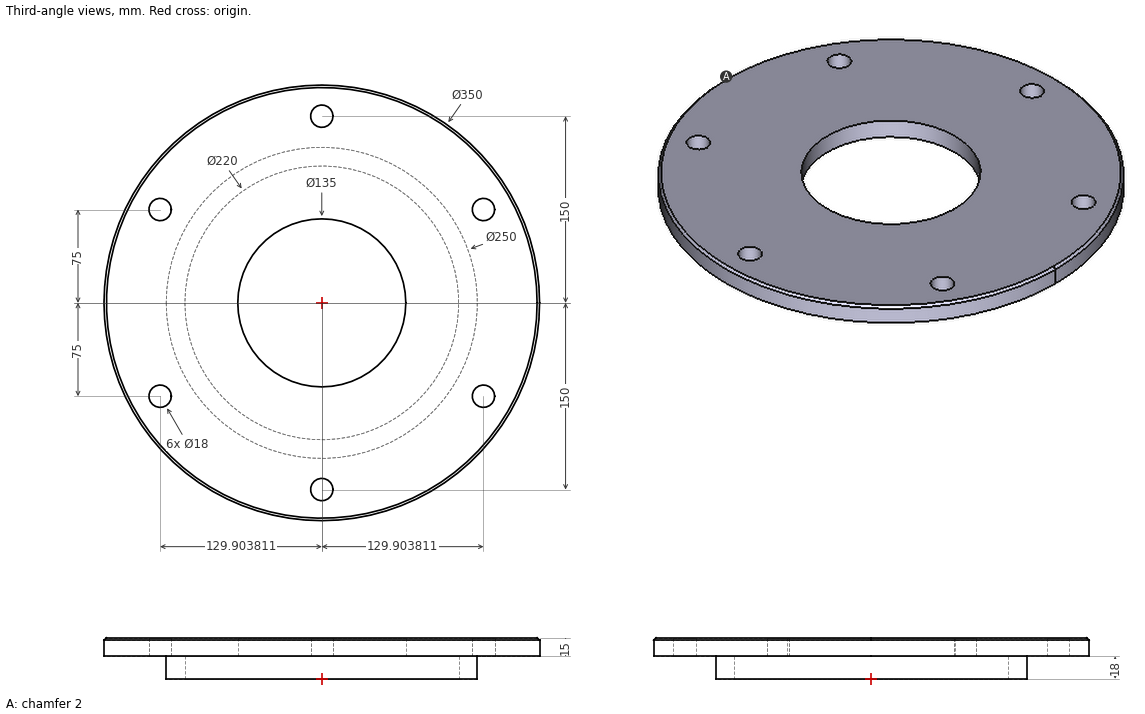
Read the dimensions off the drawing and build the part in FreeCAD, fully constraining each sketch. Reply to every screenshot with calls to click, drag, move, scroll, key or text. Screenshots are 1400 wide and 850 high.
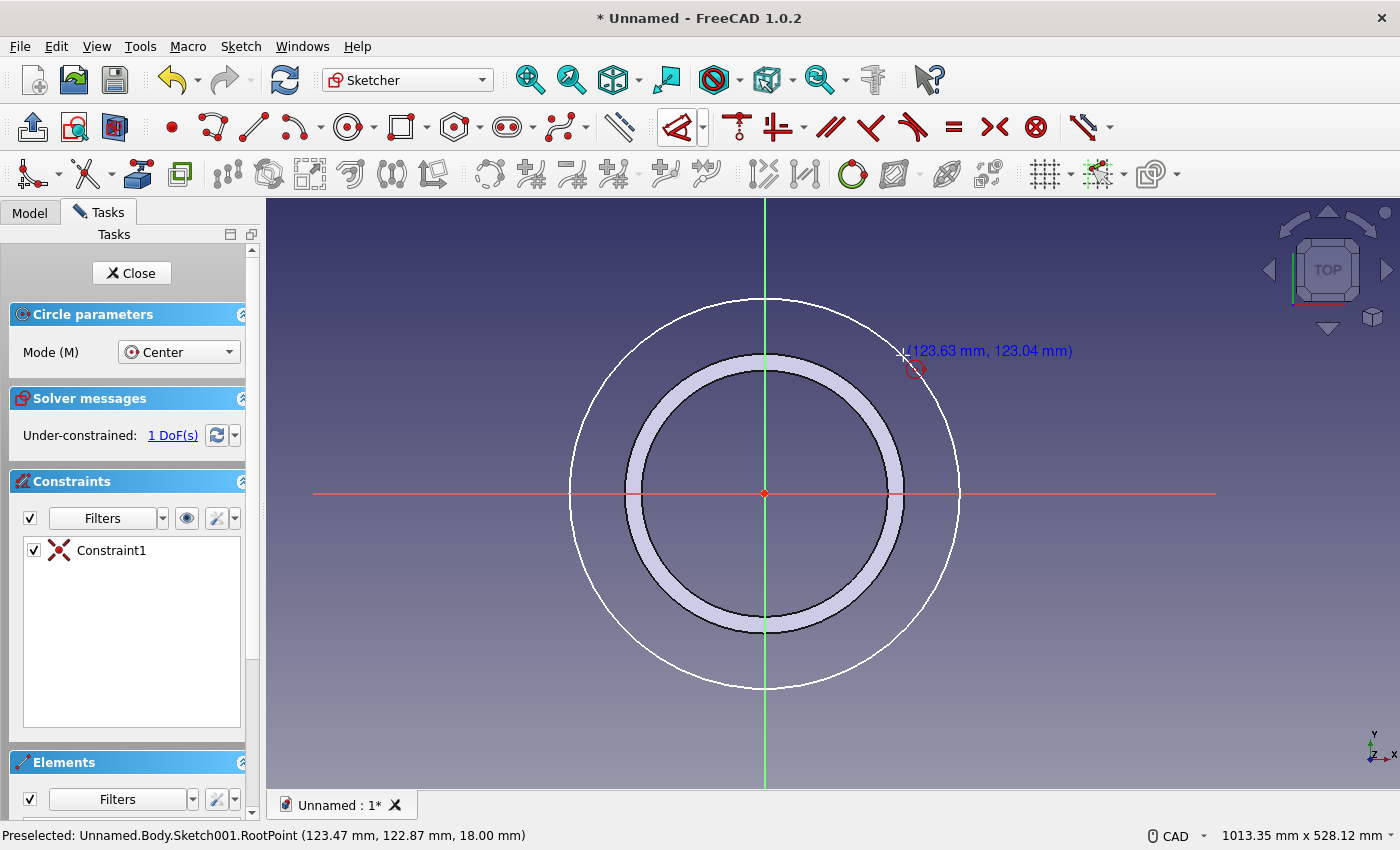
scroll(619, 578, up, 5)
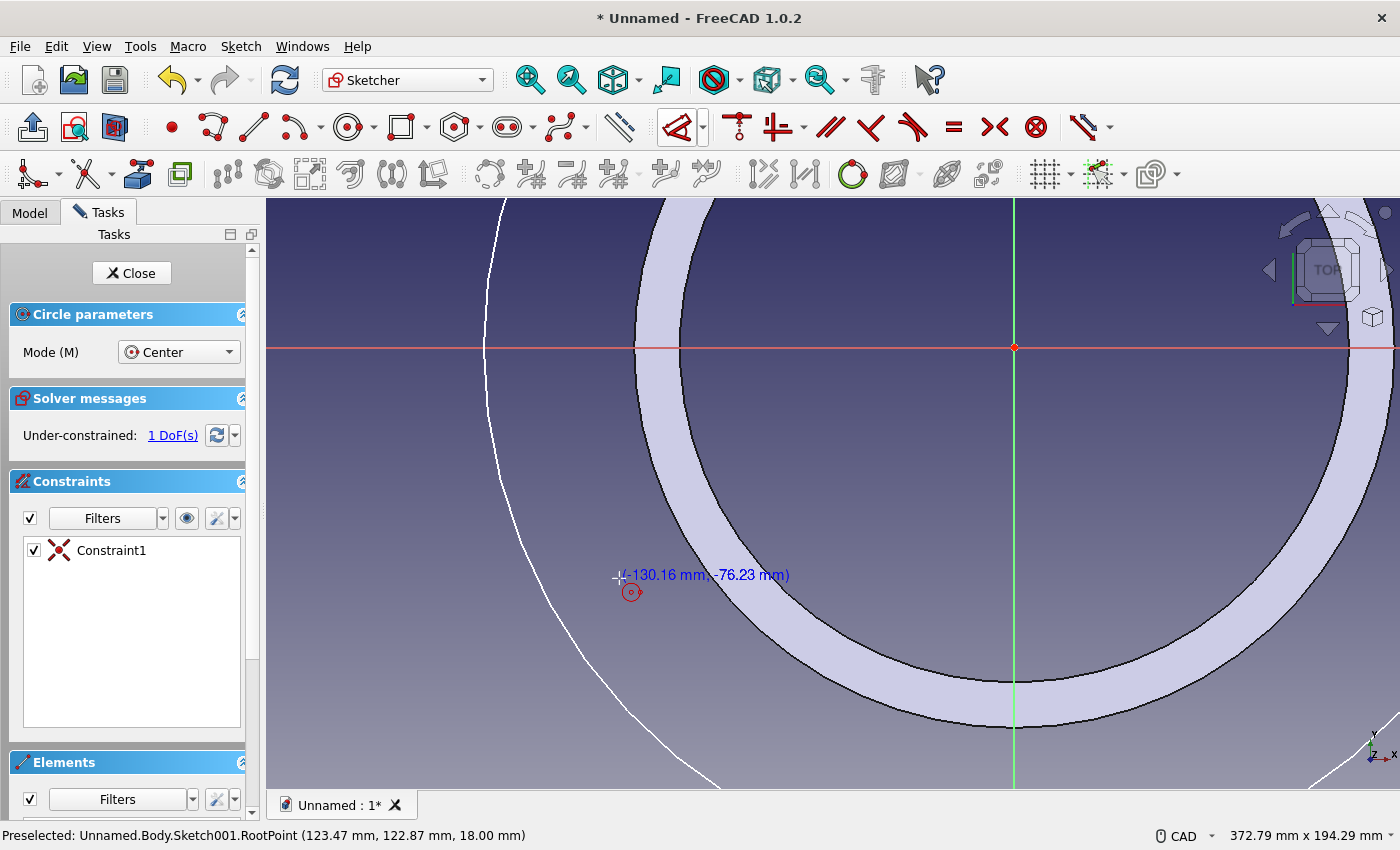
click(619, 576)
click(639, 557)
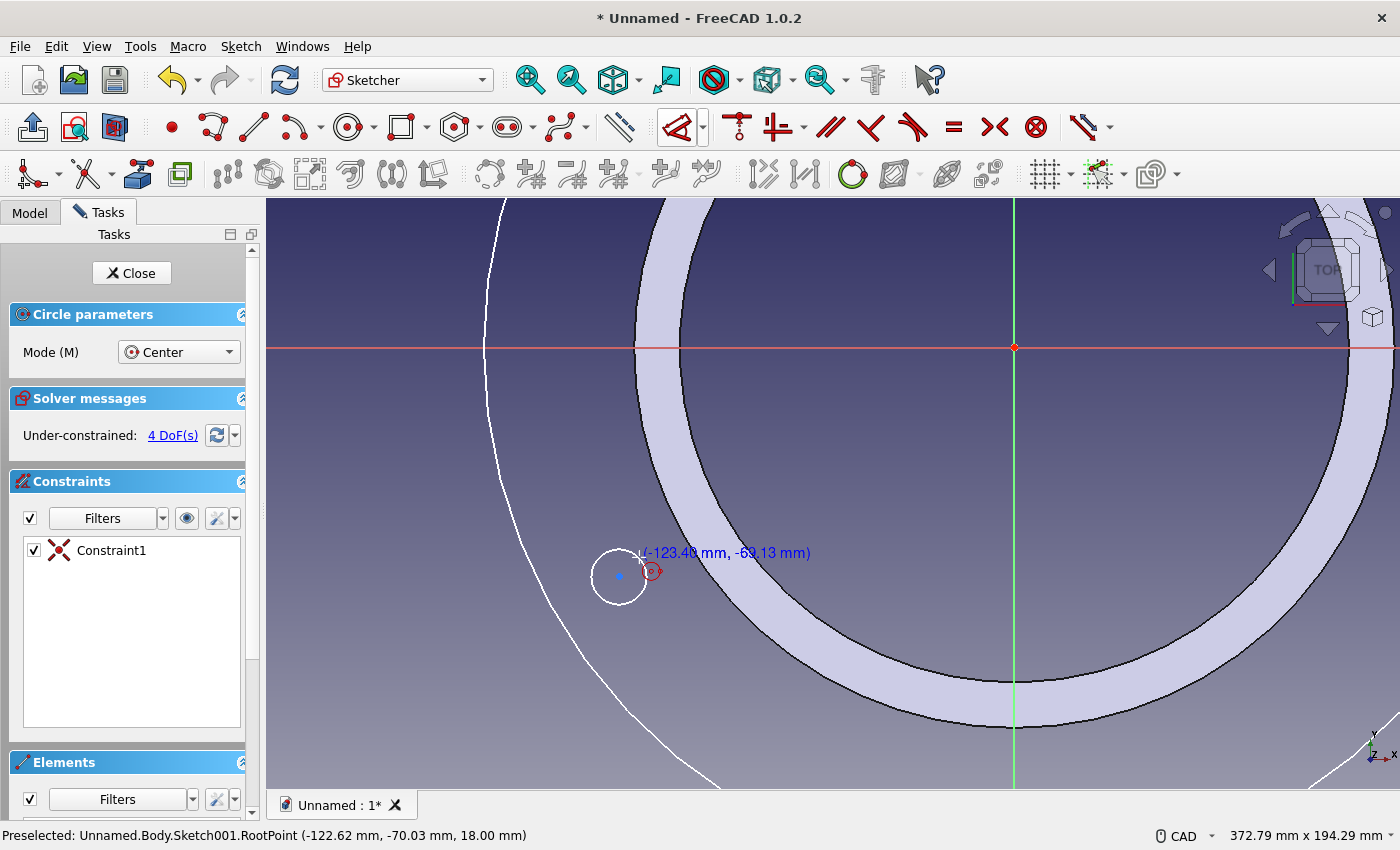
scroll(619, 578, down, 5)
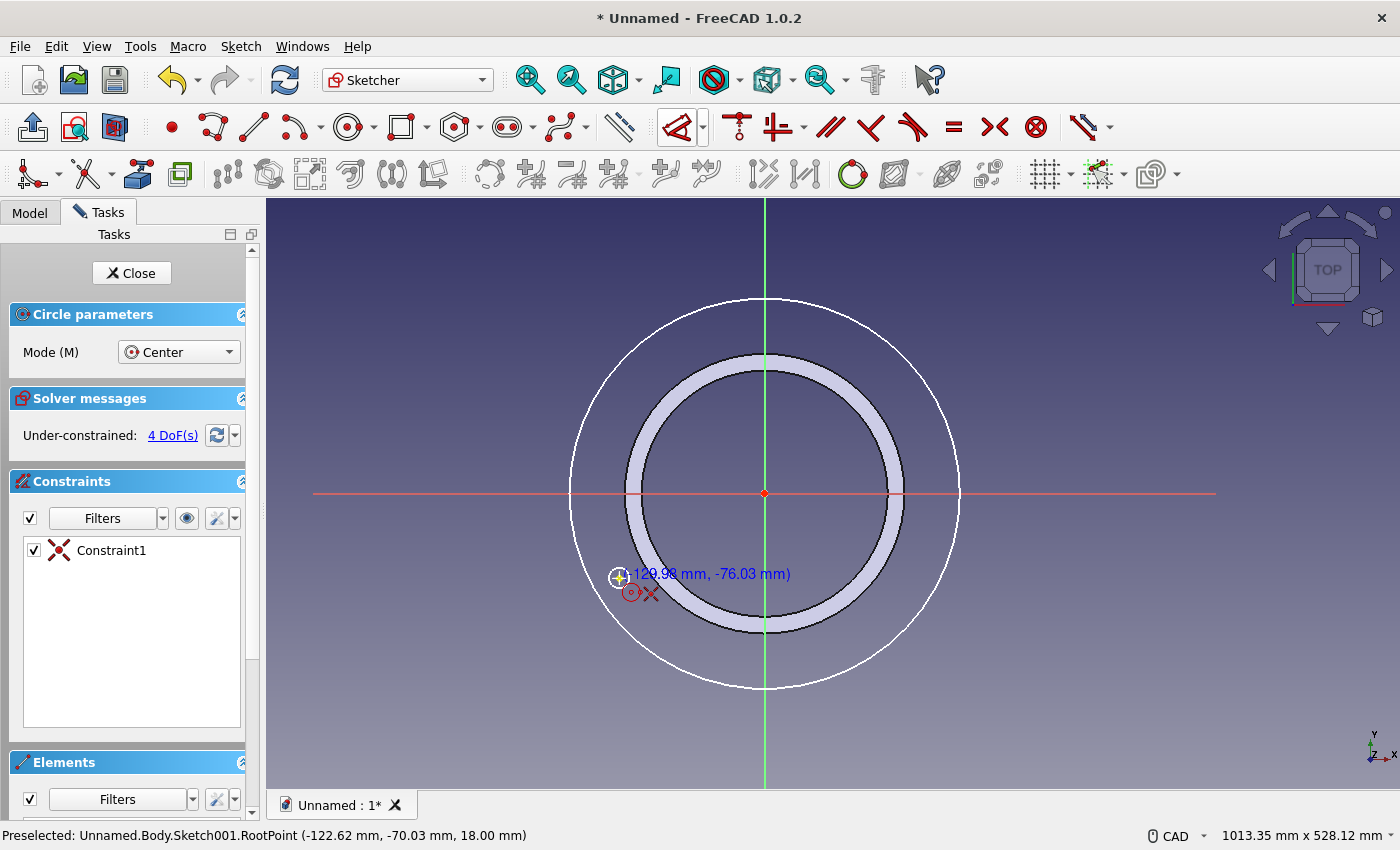
scroll(765, 662, up, 5)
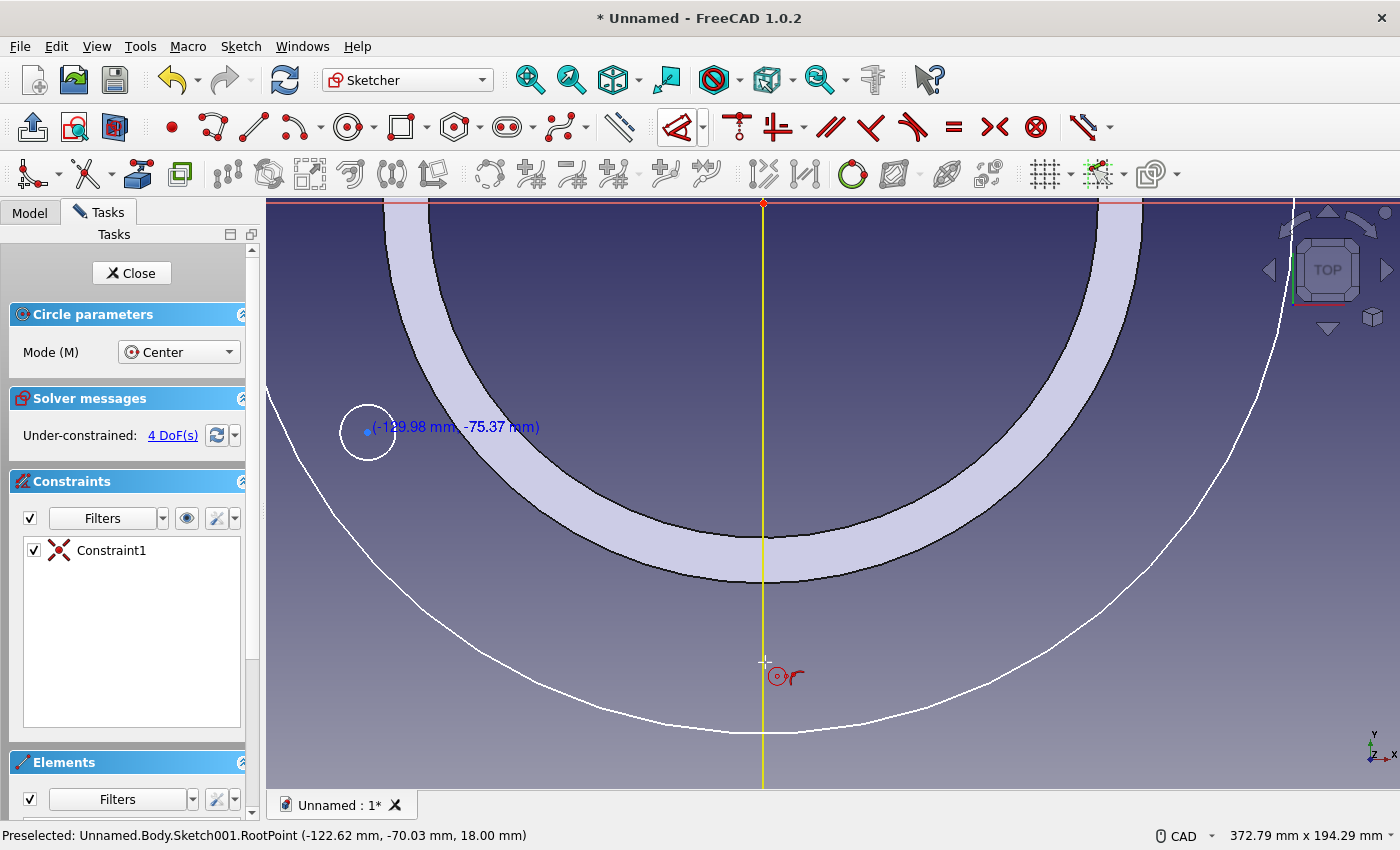
click(763, 659)
click(783, 640)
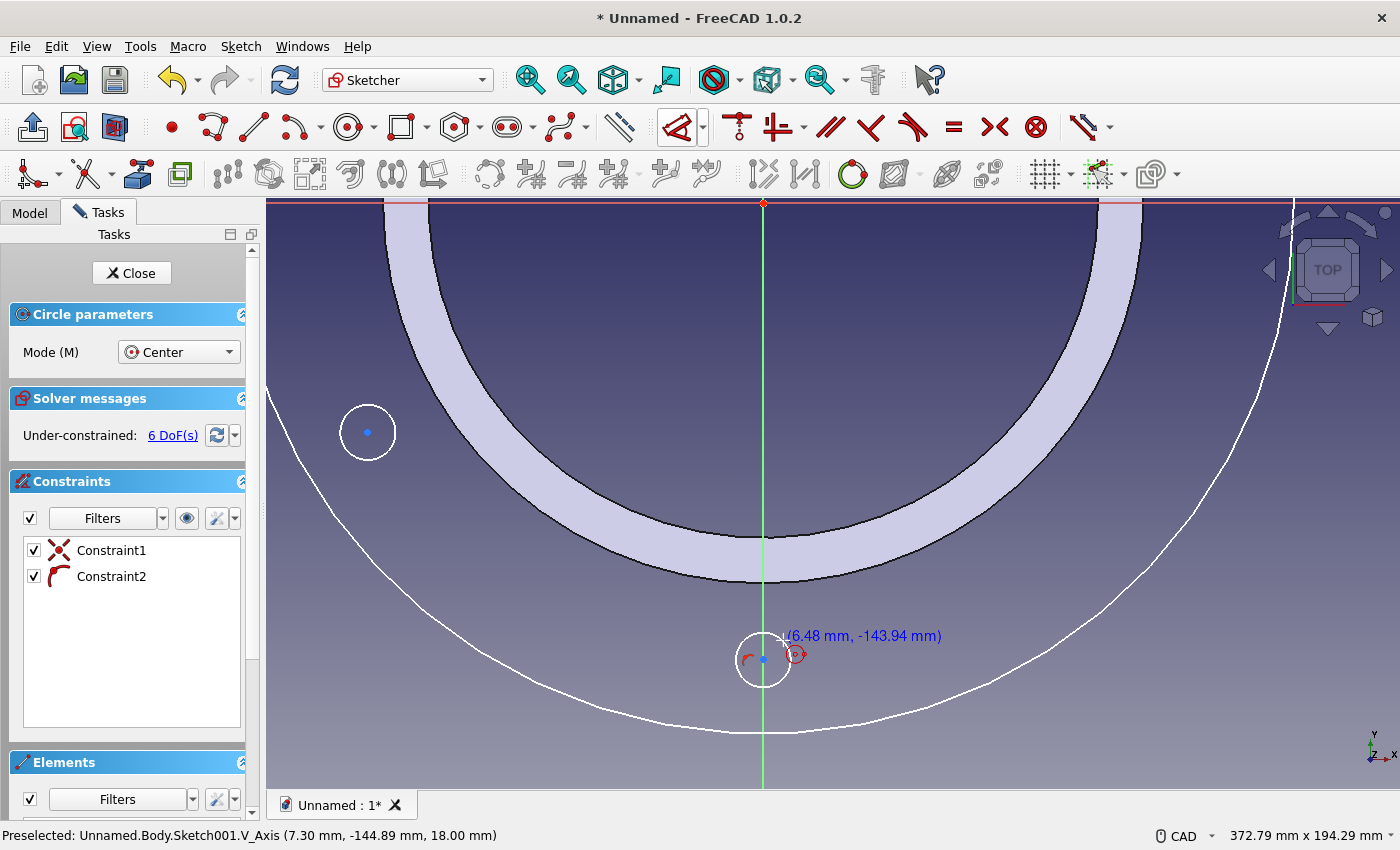
click(1158, 431)
click(1178, 412)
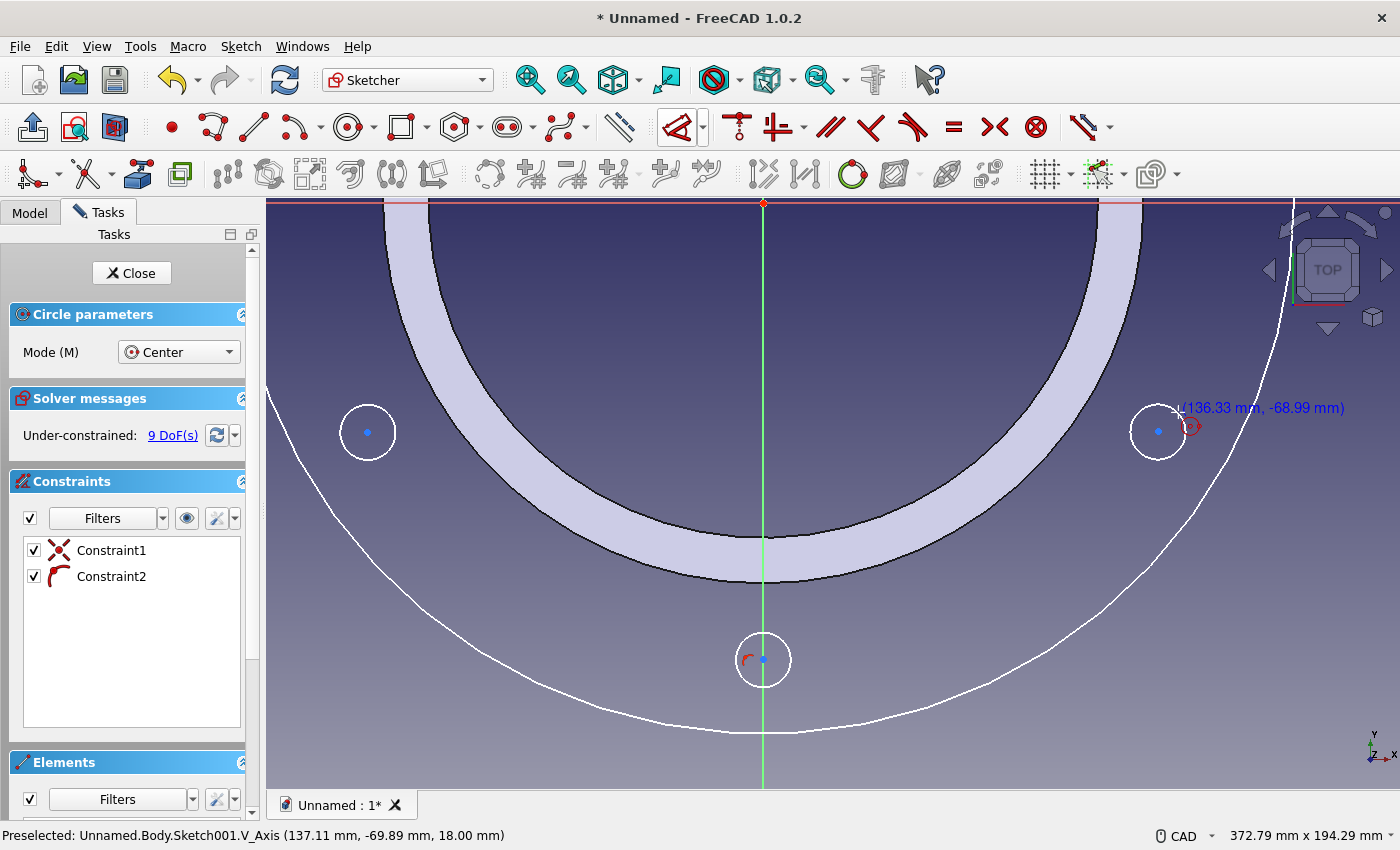
scroll(765, 662, down, 5)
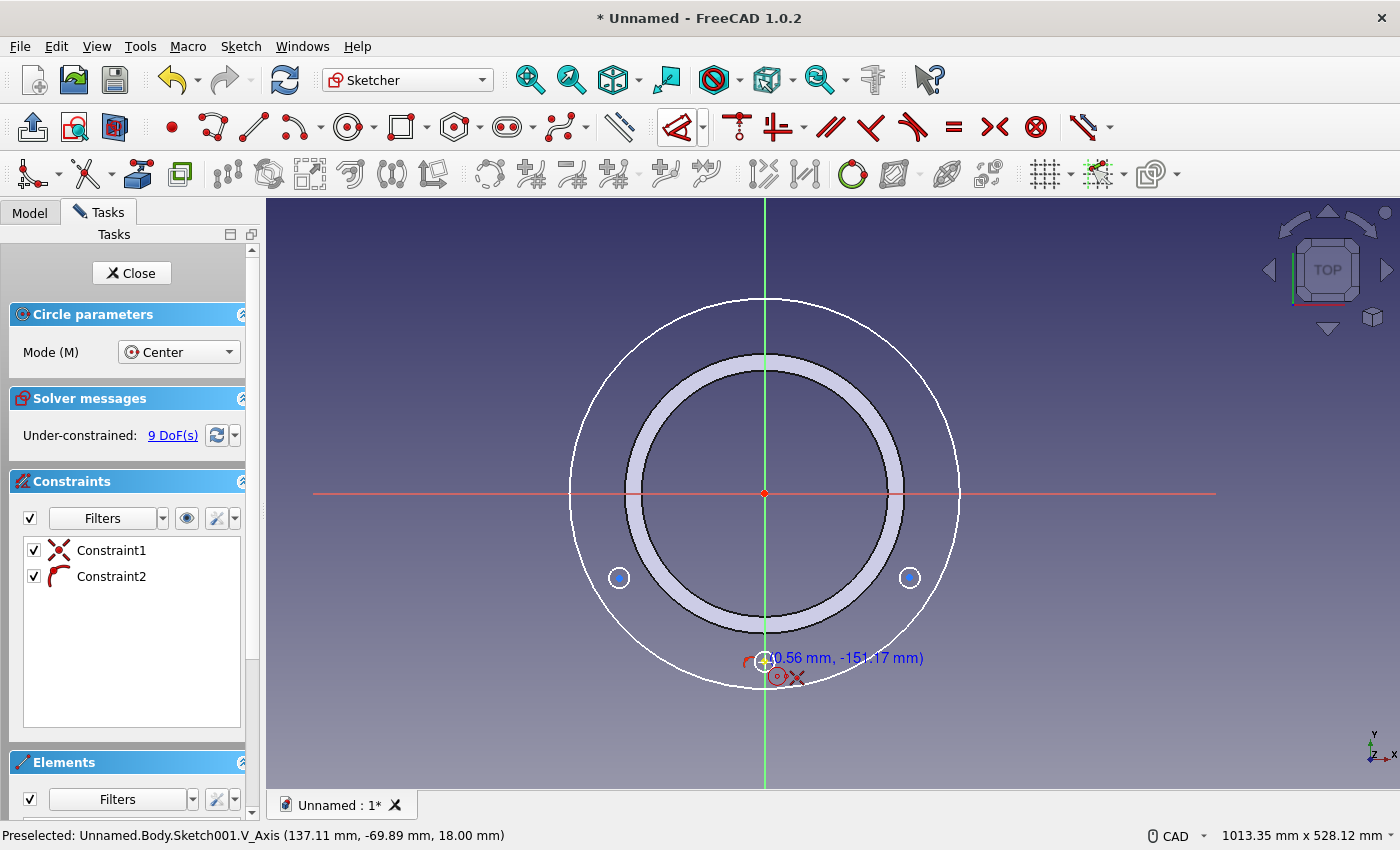
scroll(619, 410, up, 5)